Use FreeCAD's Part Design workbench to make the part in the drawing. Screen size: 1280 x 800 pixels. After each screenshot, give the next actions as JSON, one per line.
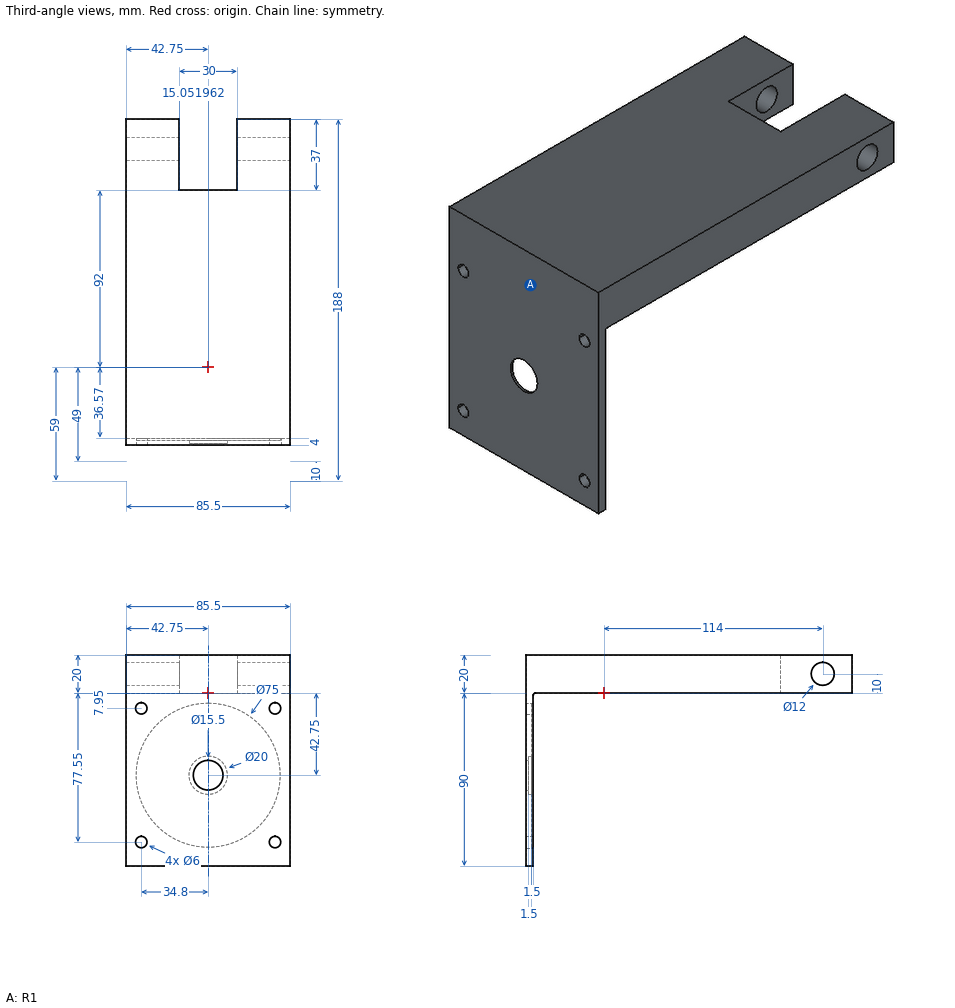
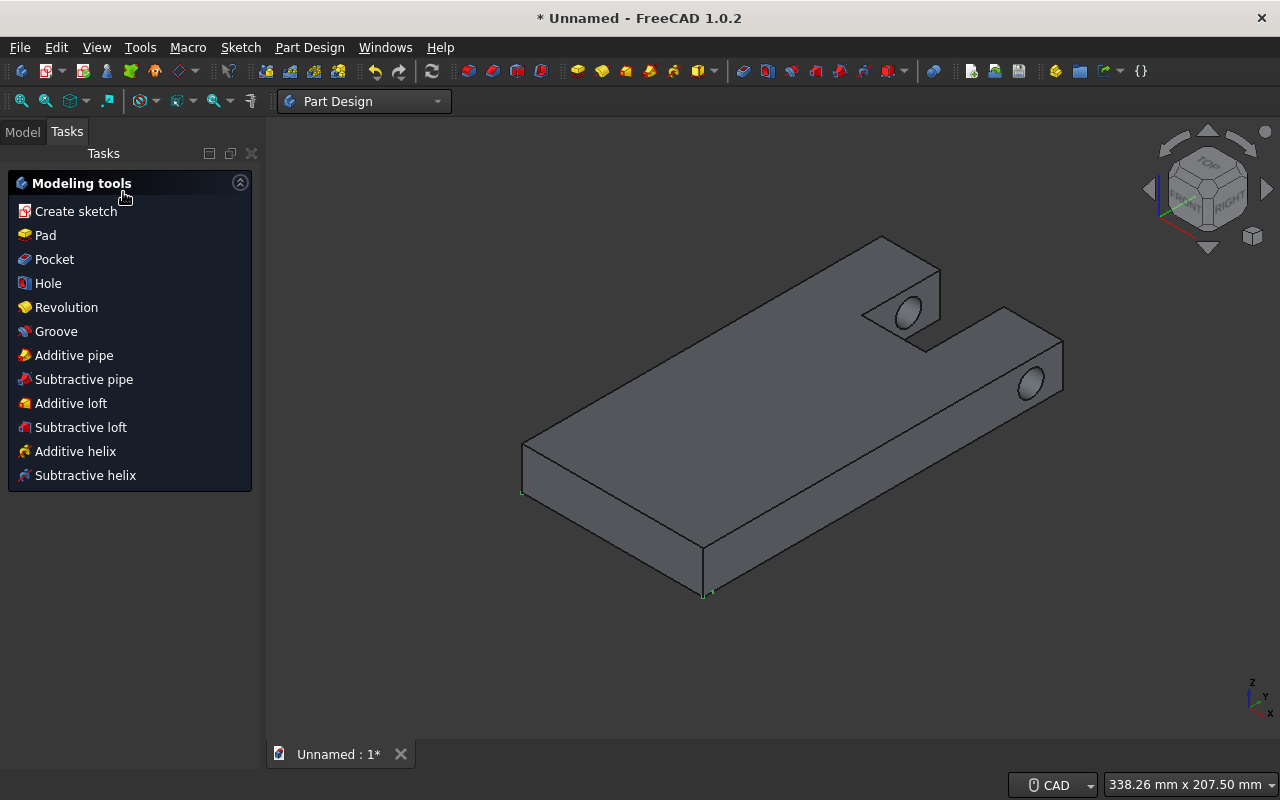
{"action": "left_click", "coordinate": [578, 72]}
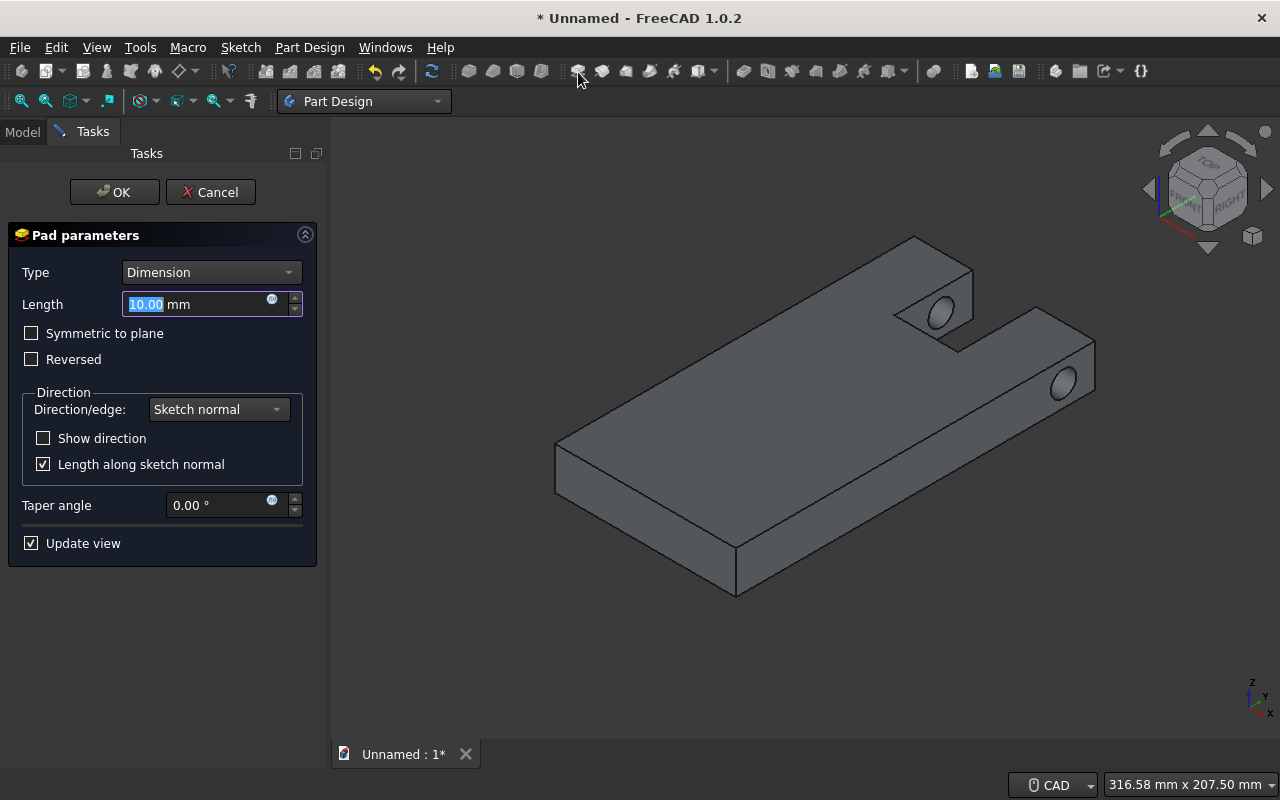
{"action": "type", "text": "90"}
{"action": "key", "text": "Tab"}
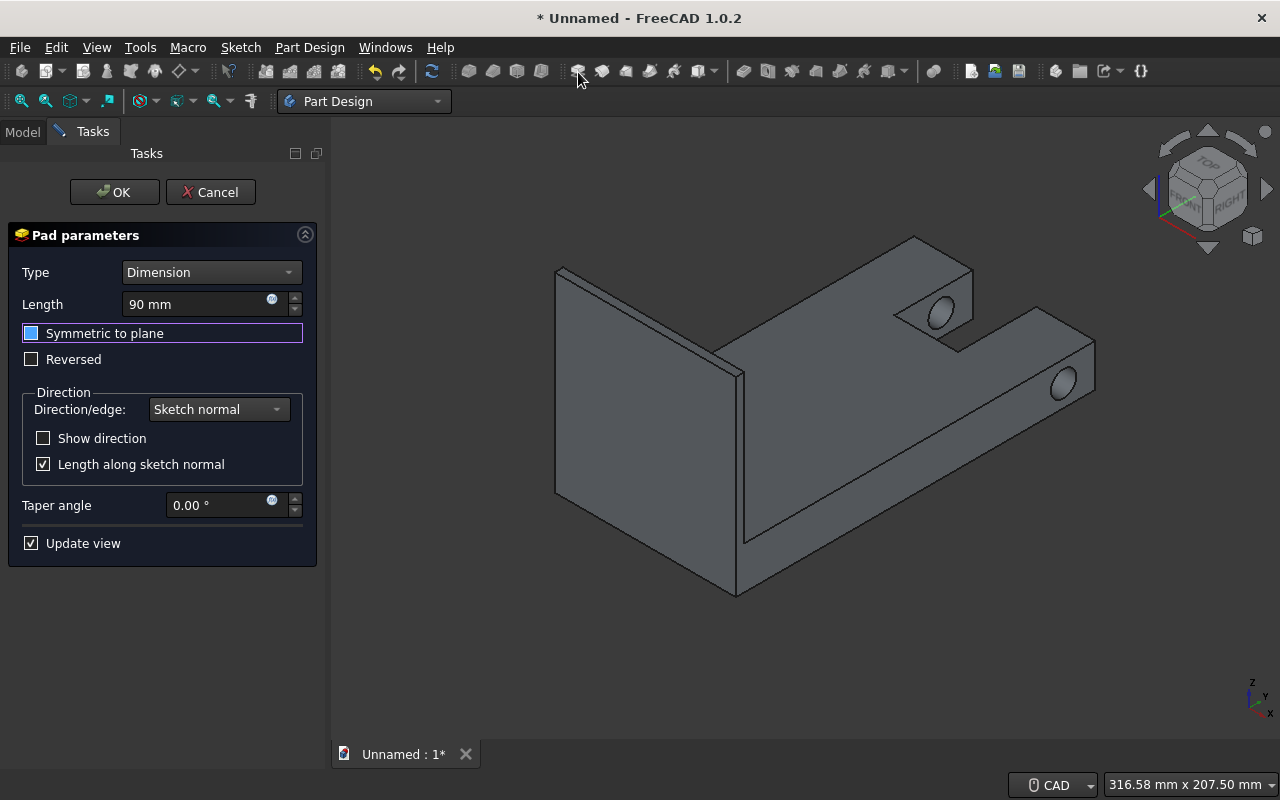
{"action": "left_click", "coordinate": [30, 359]}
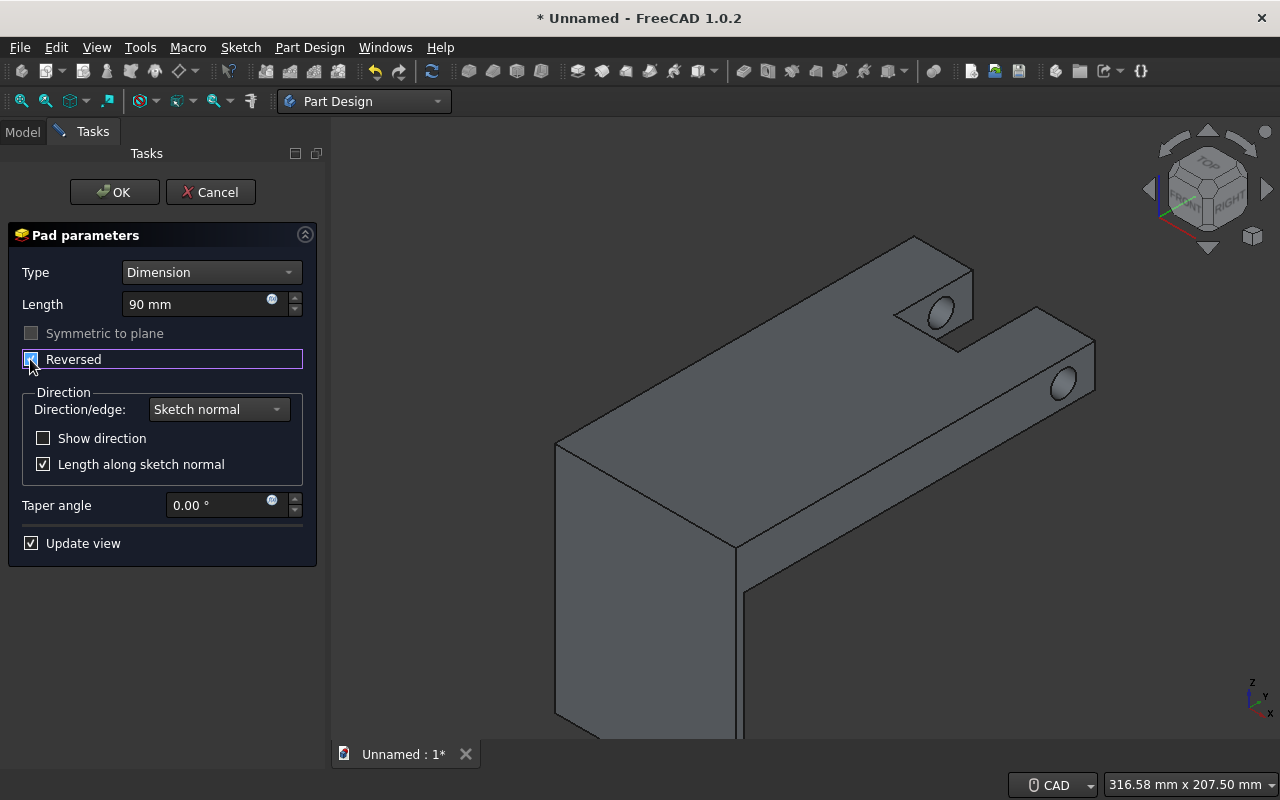
{"action": "left_click", "coordinate": [115, 192]}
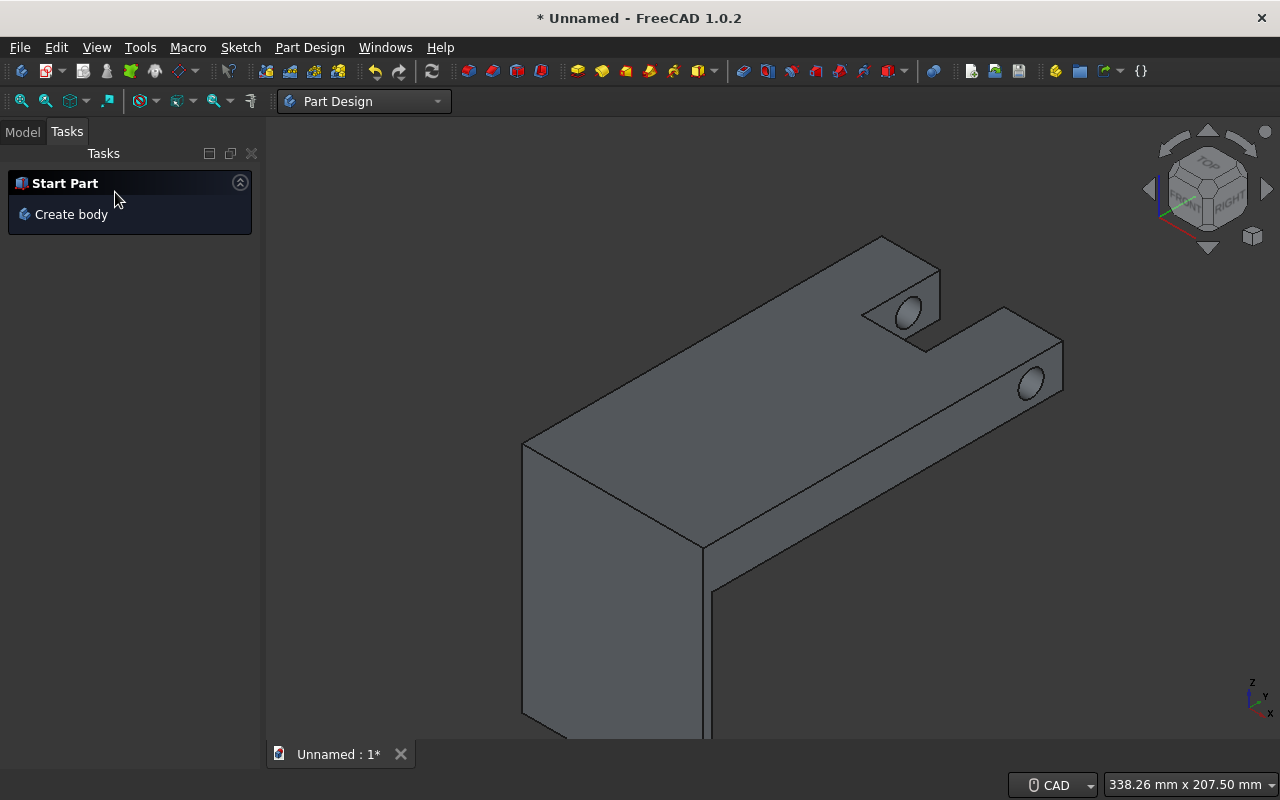
{"action": "key", "text": "v f"}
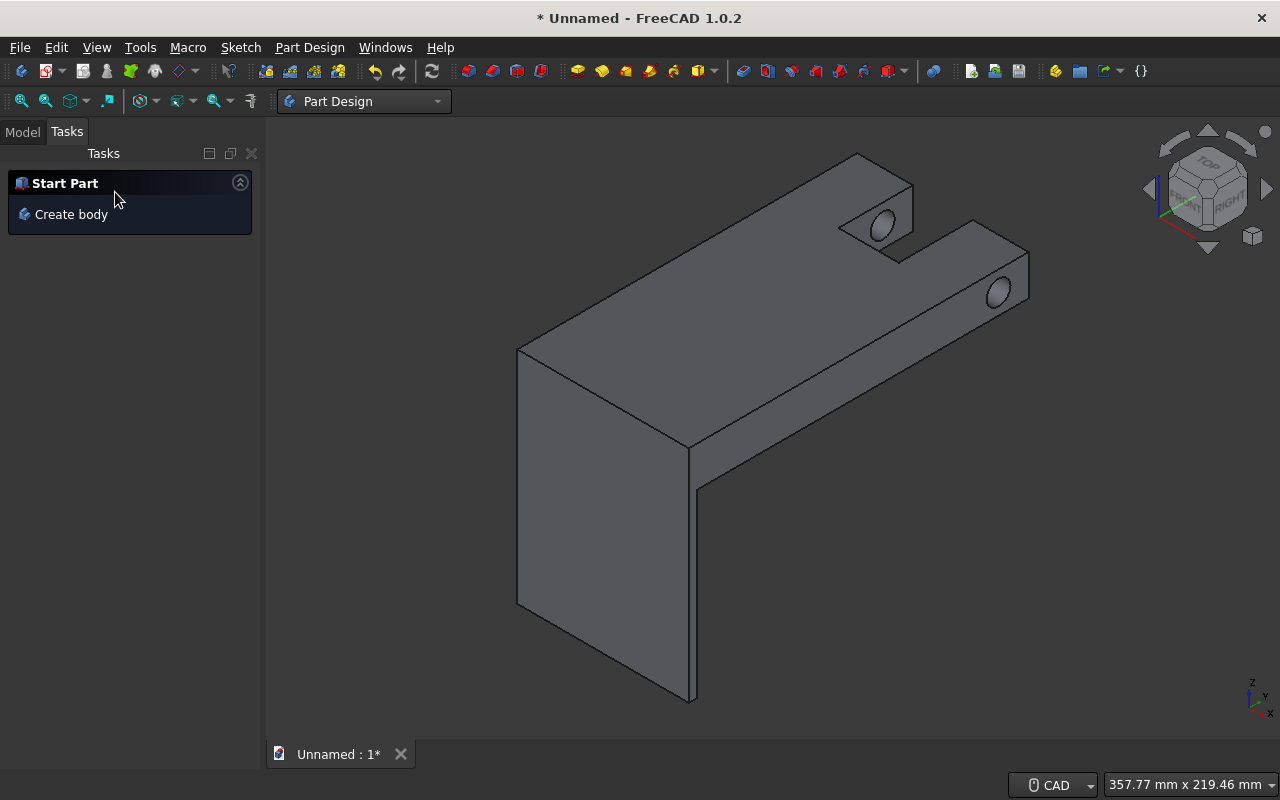
{"action": "key", "text": "4"}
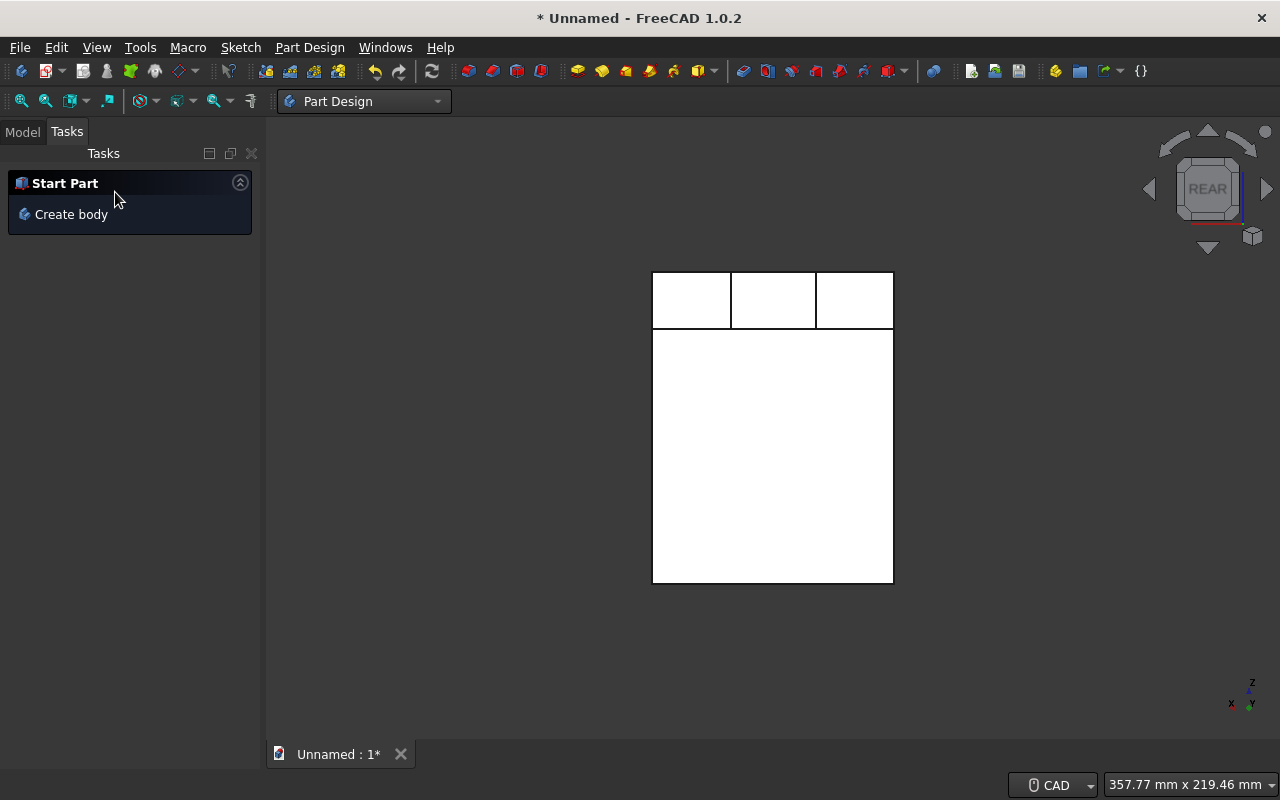
{"action": "left_click", "coordinate": [773, 455]}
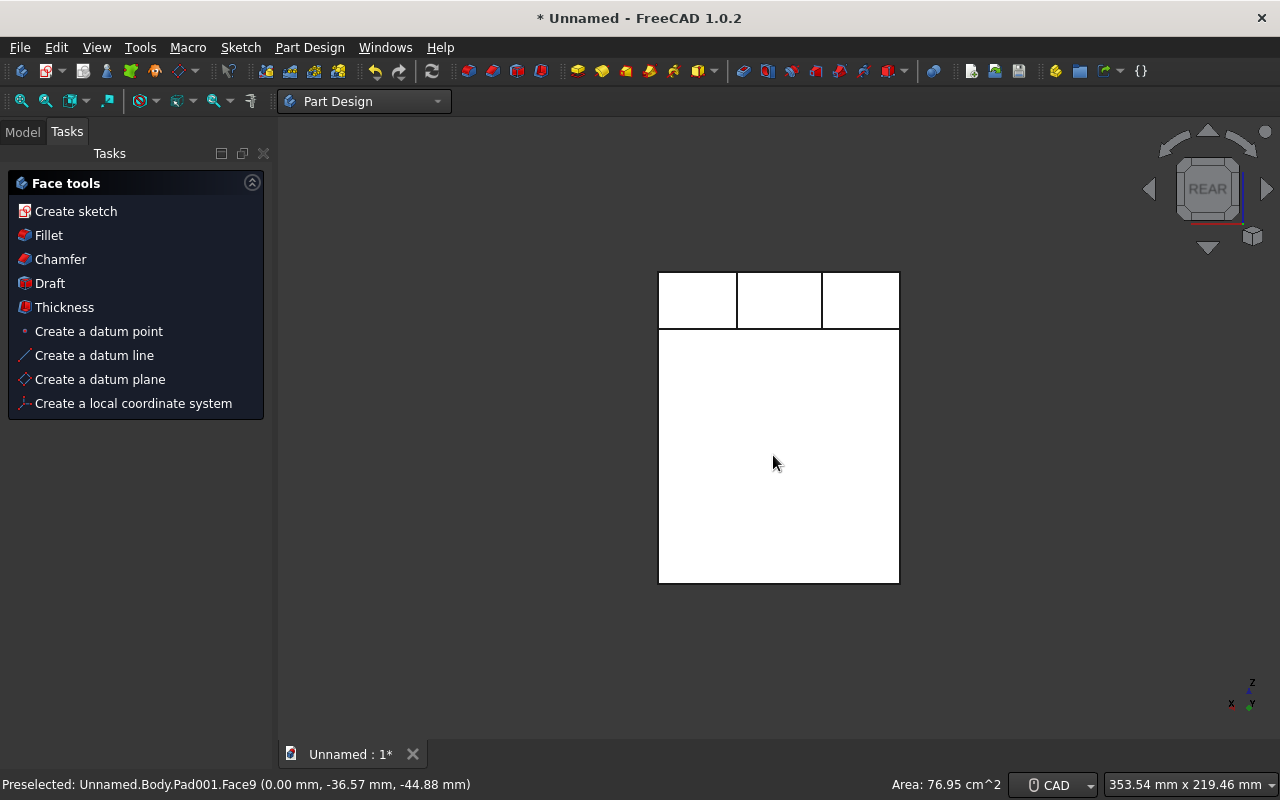
{"action": "left_click", "coordinate": [46, 72]}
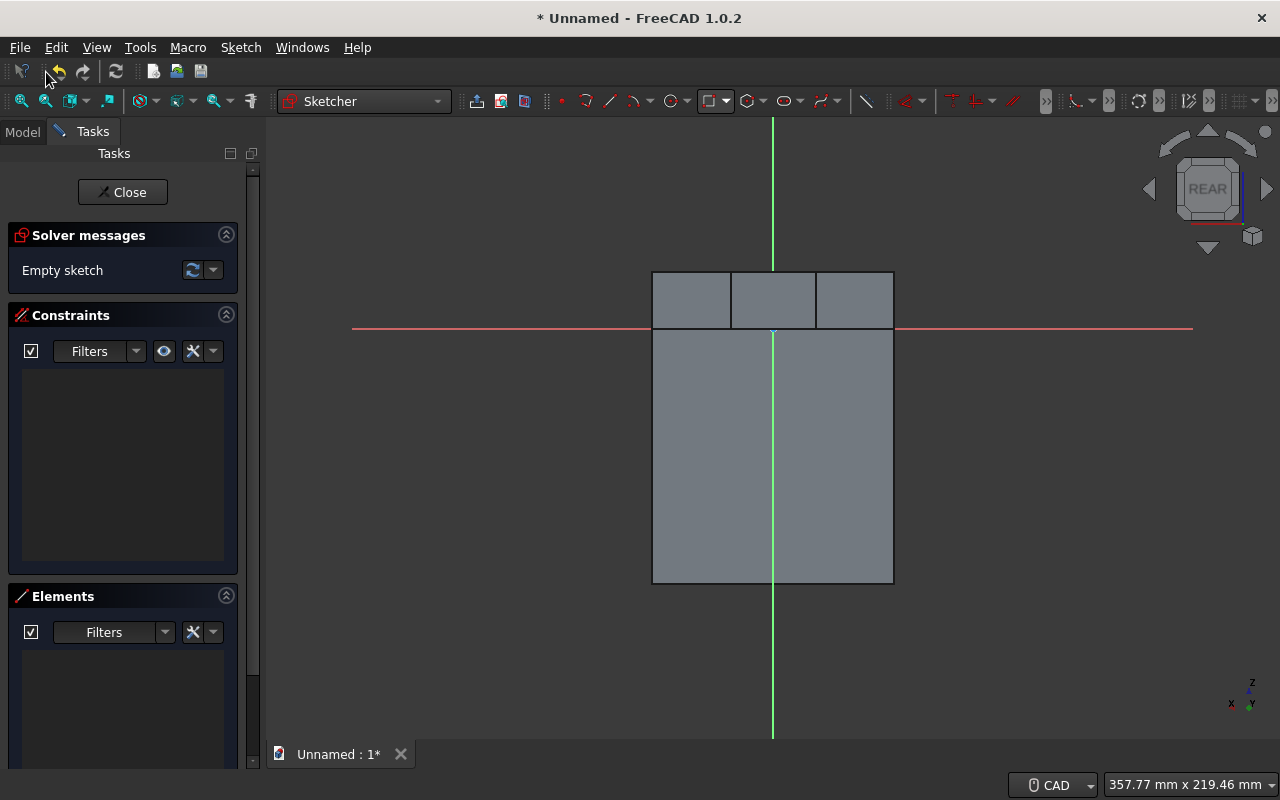
{"action": "scroll", "coordinate": [856, 461], "scroll_direction": "up", "scroll_amount": 3}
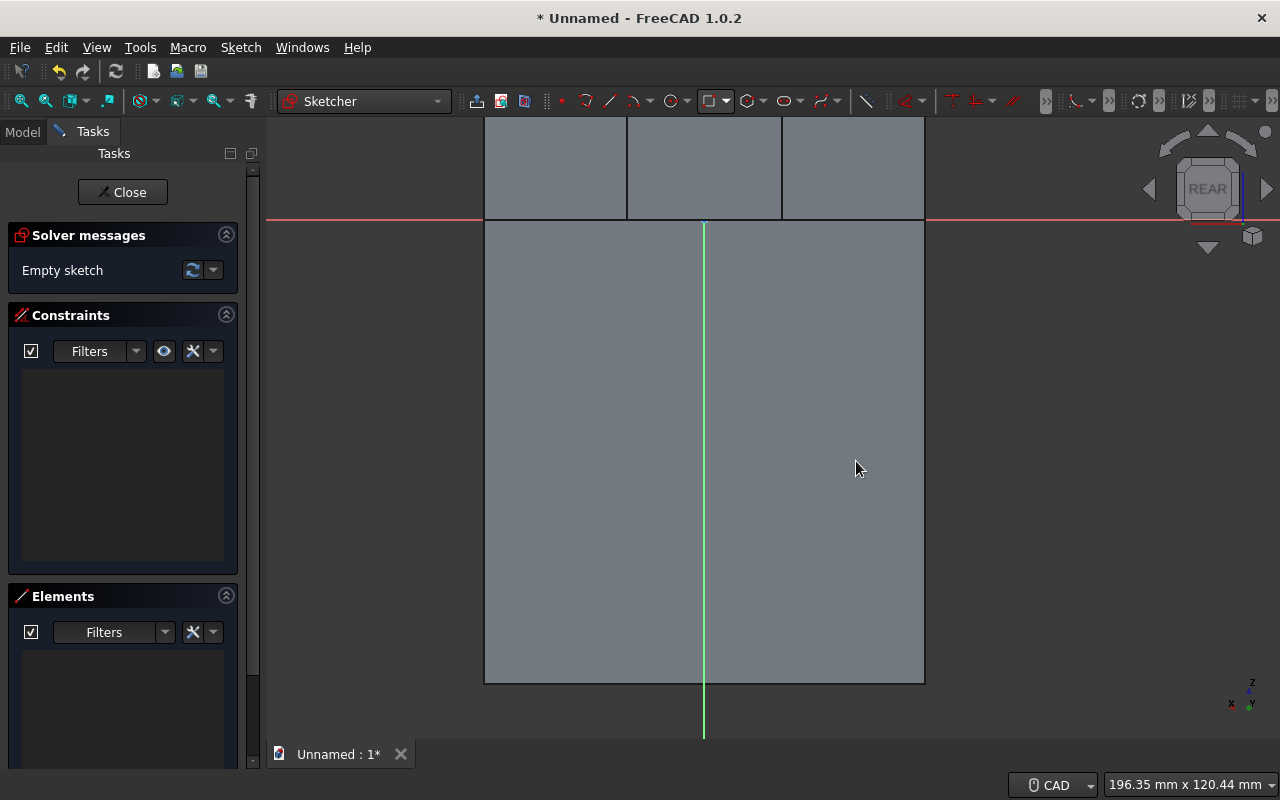
{"action": "left_click", "coordinate": [672, 102]}